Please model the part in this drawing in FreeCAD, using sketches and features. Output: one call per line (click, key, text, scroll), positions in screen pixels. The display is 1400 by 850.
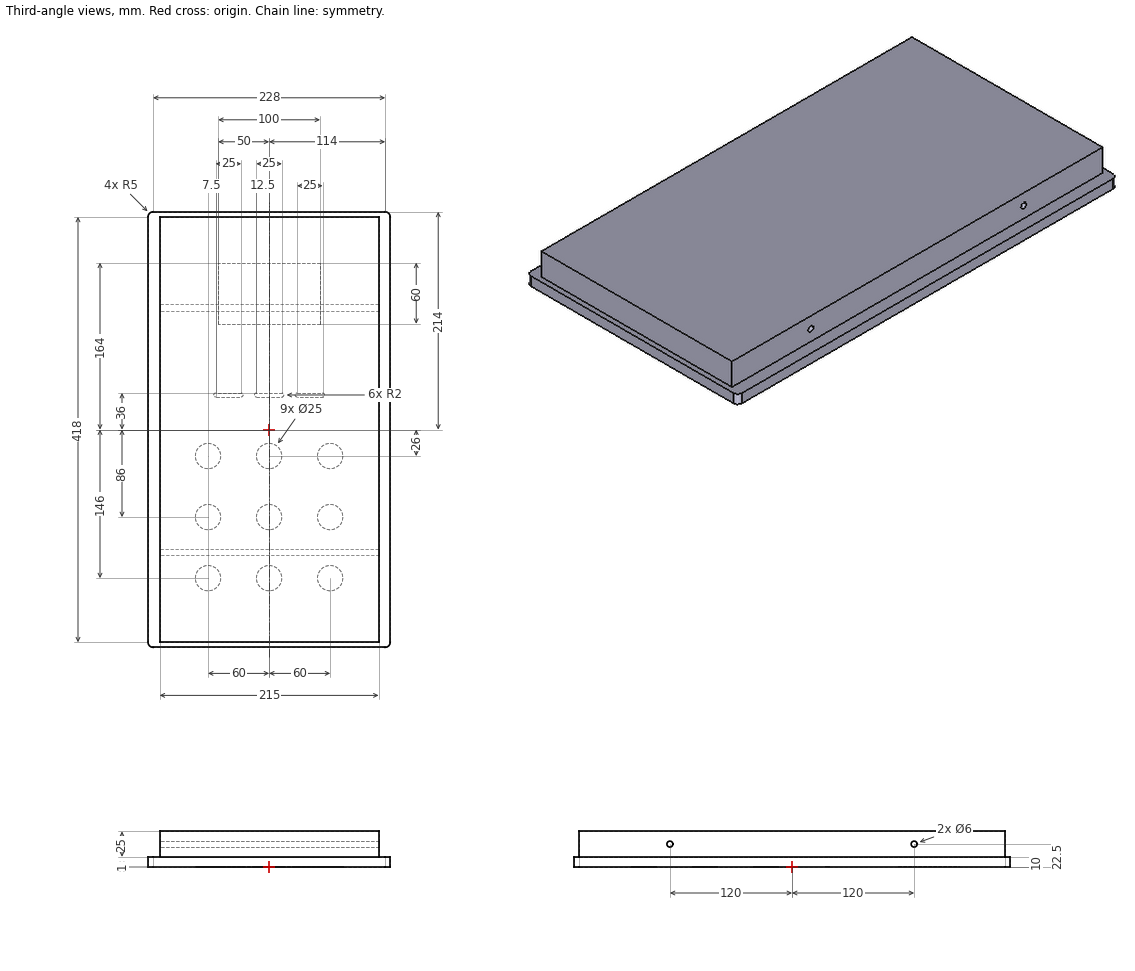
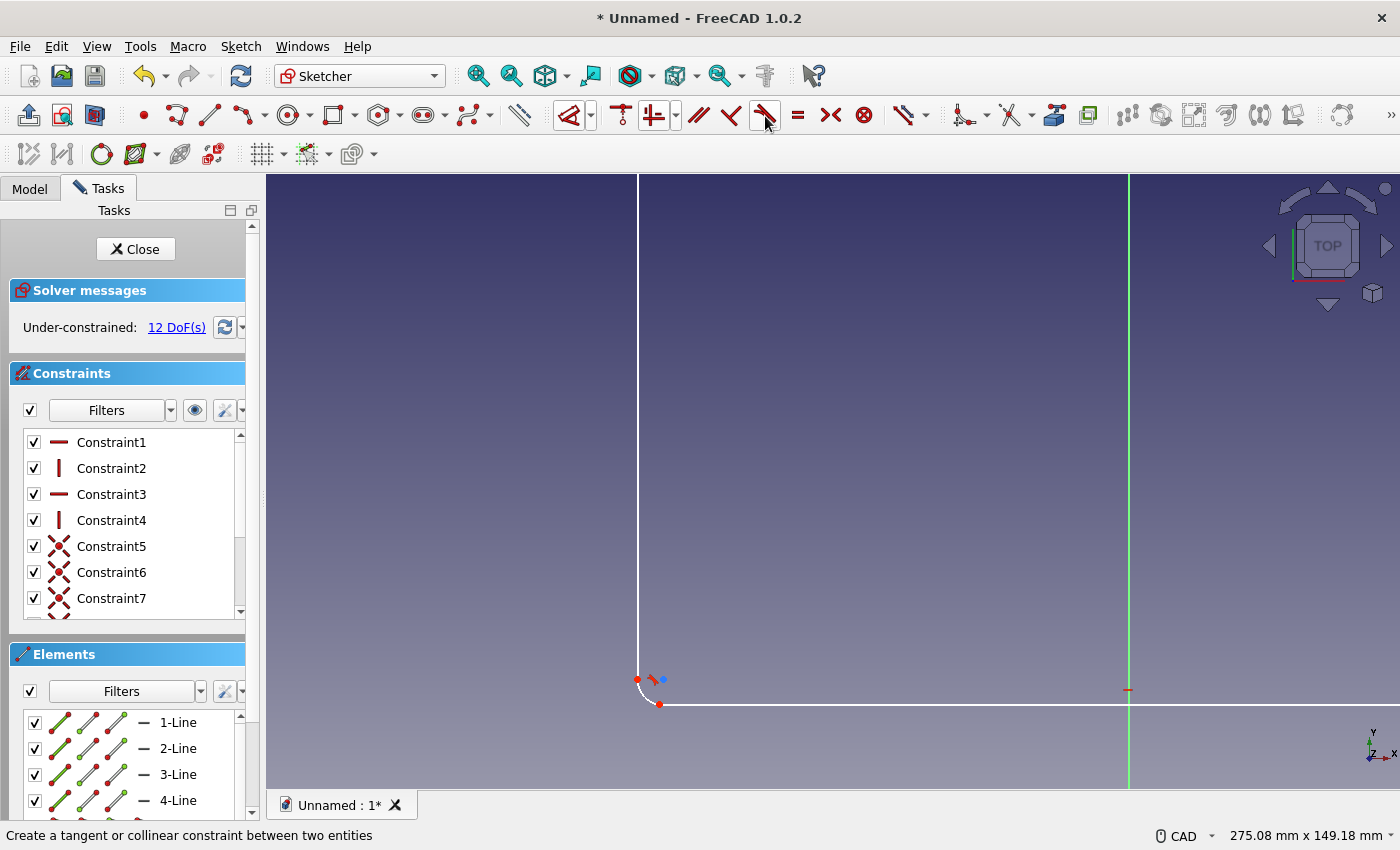
scroll(645, 698, down, 7)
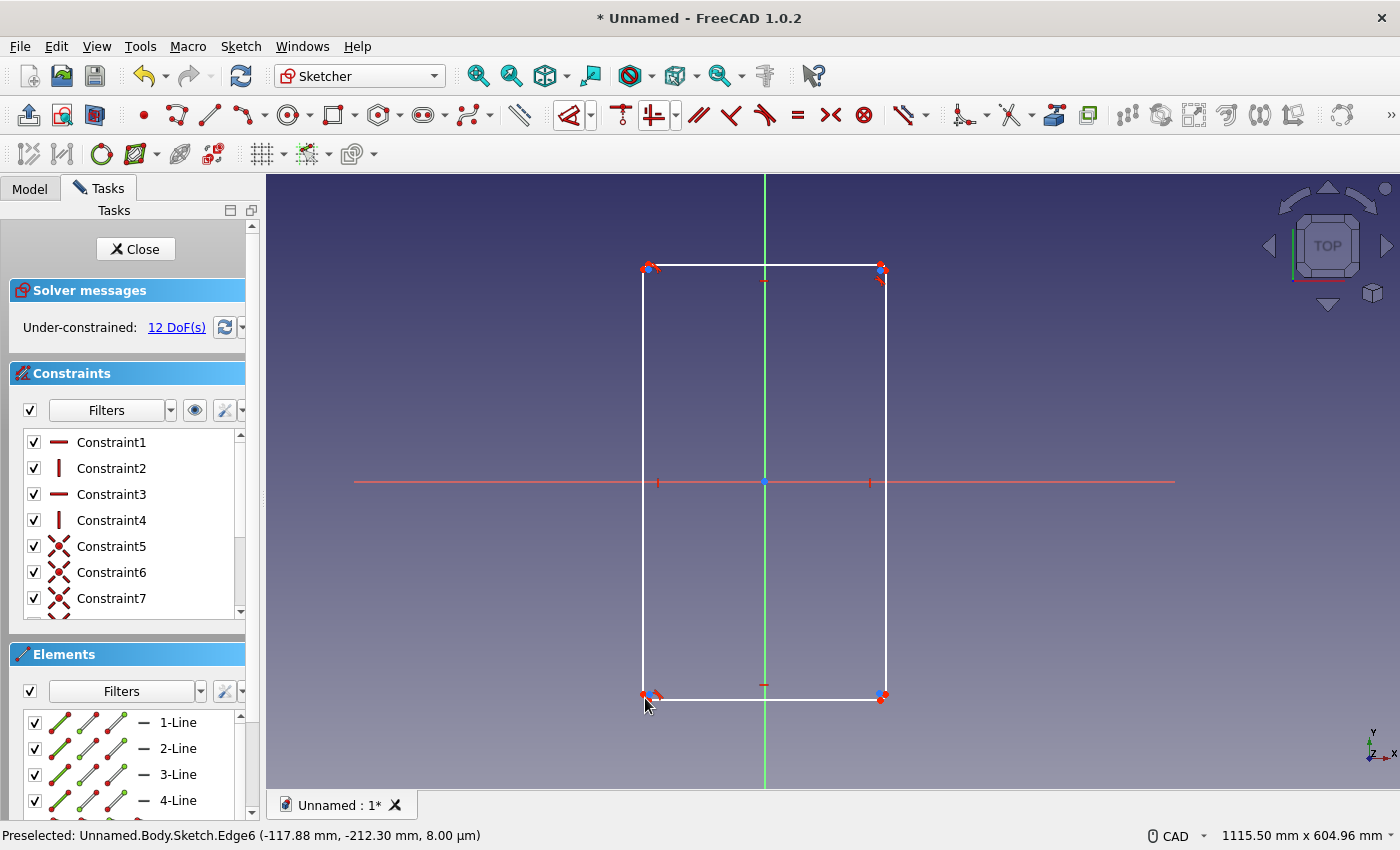
click(718, 700)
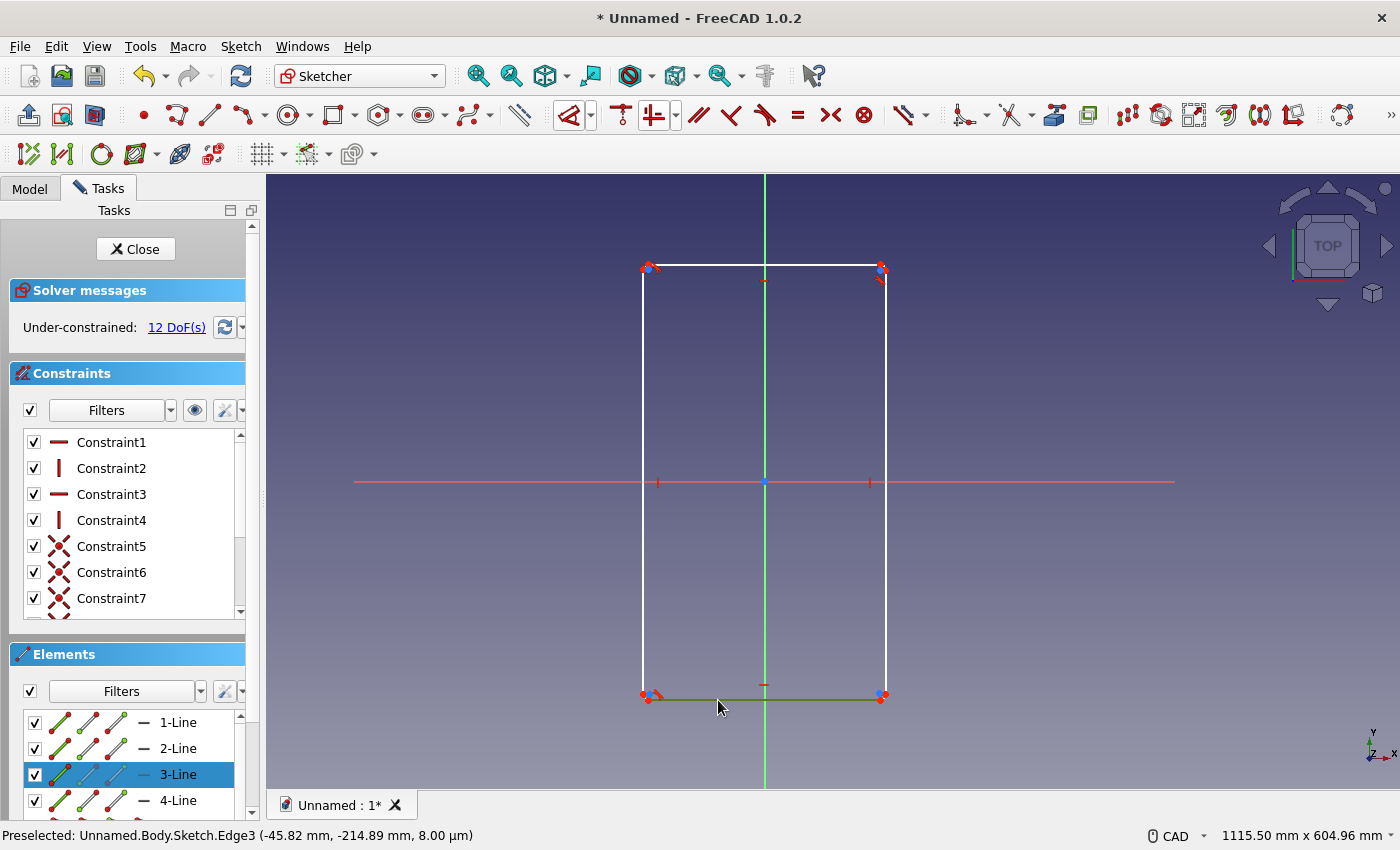
scroll(645, 698, up, 6)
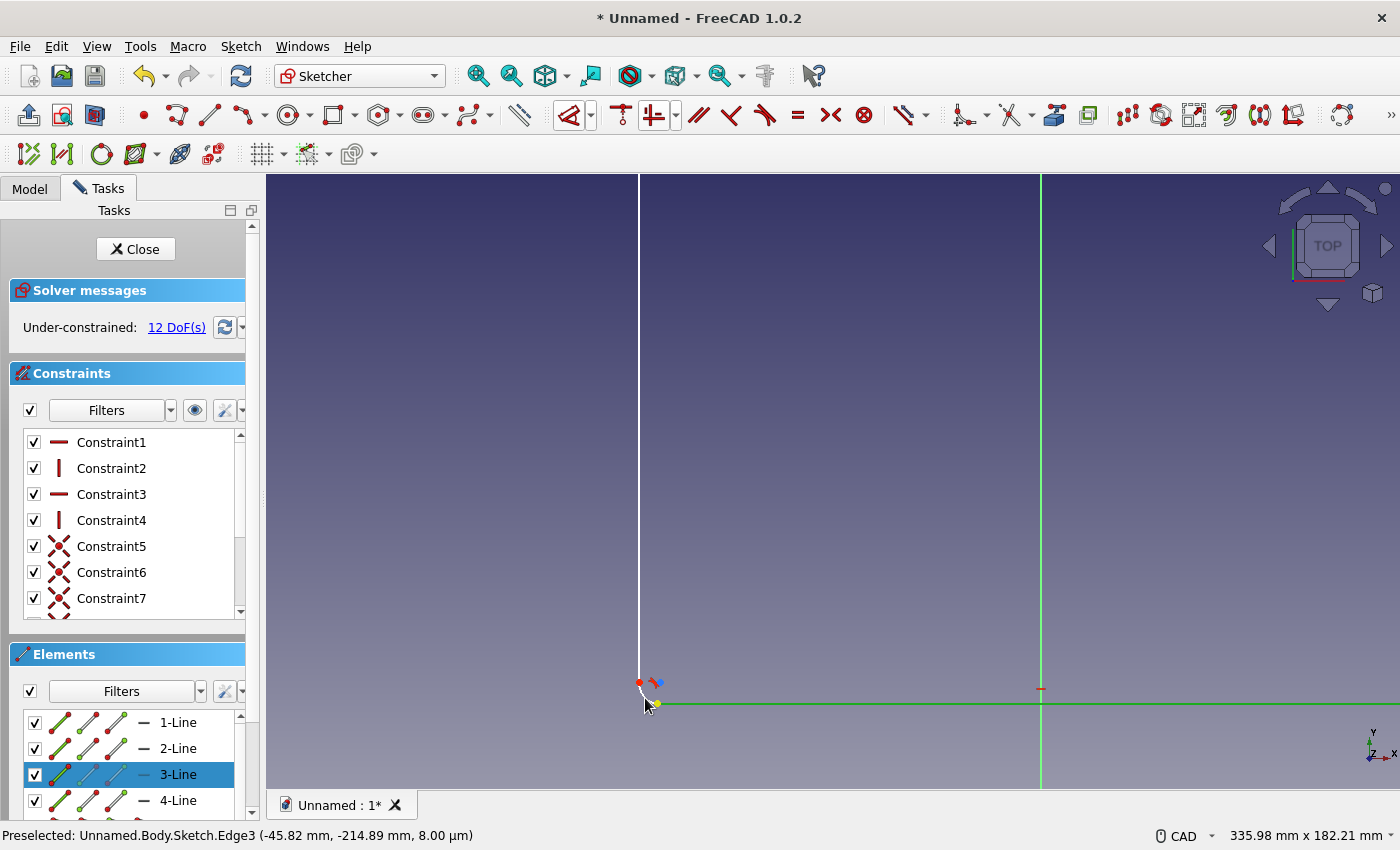
click(644, 697)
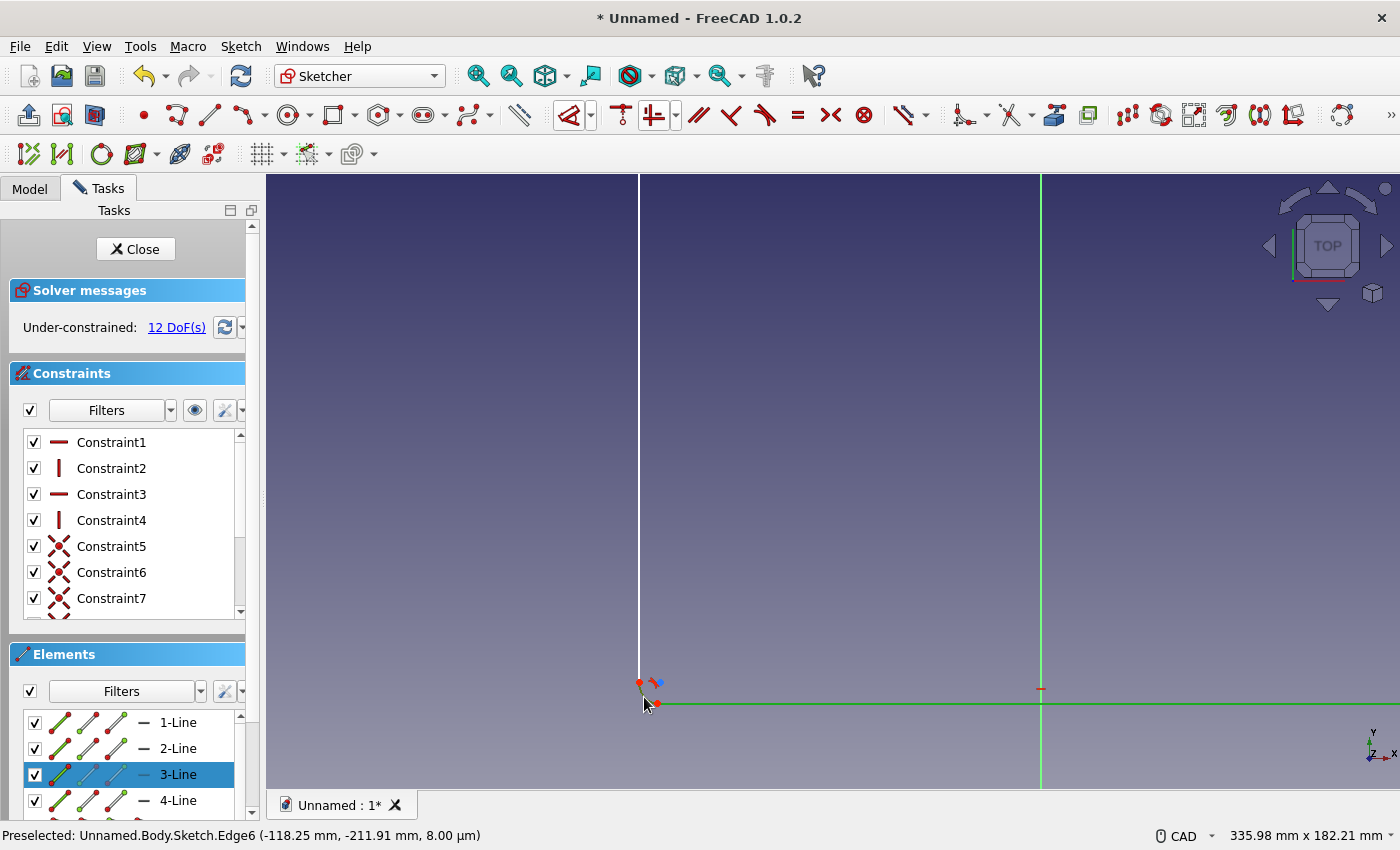
click(765, 116)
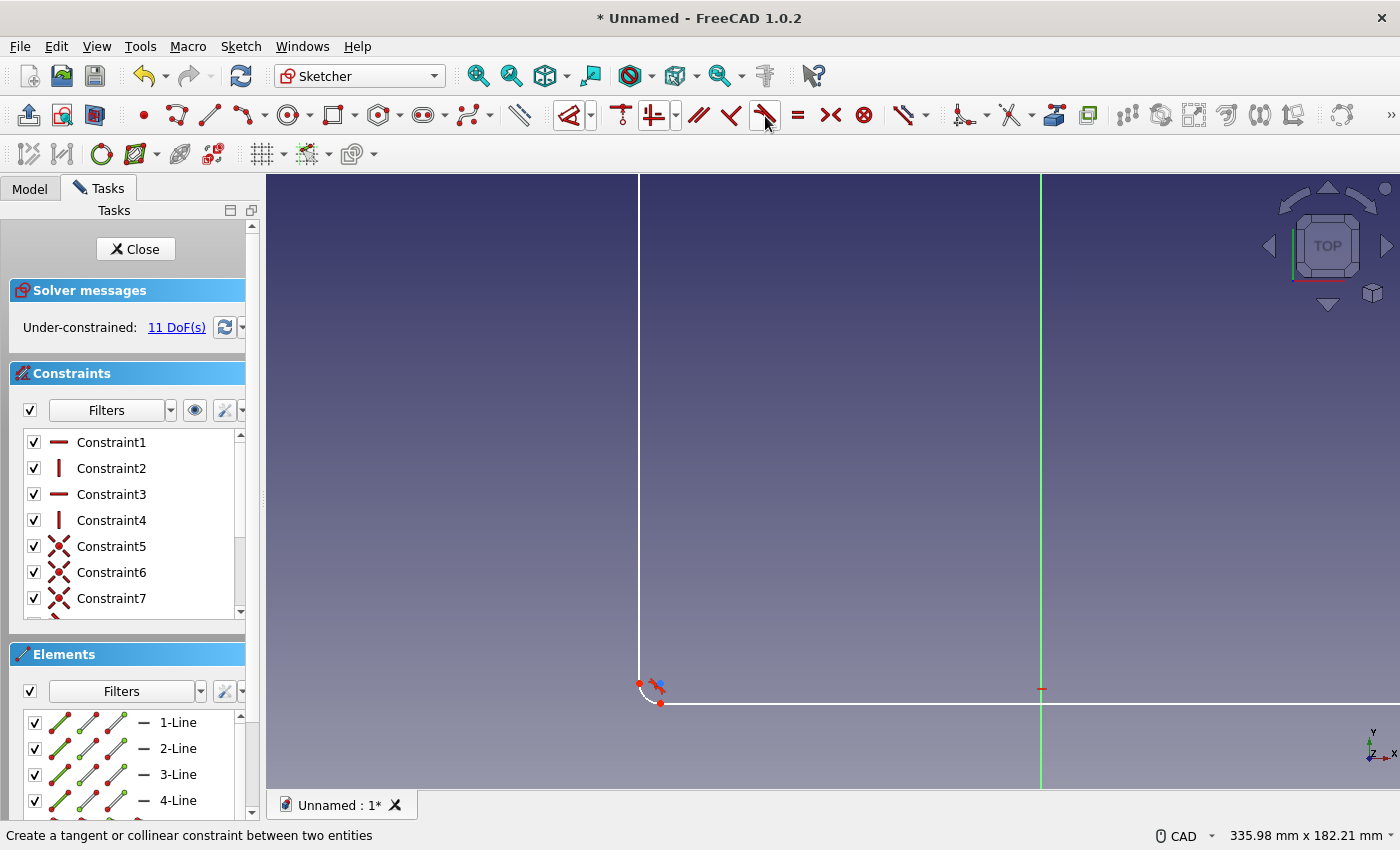
click(890, 704)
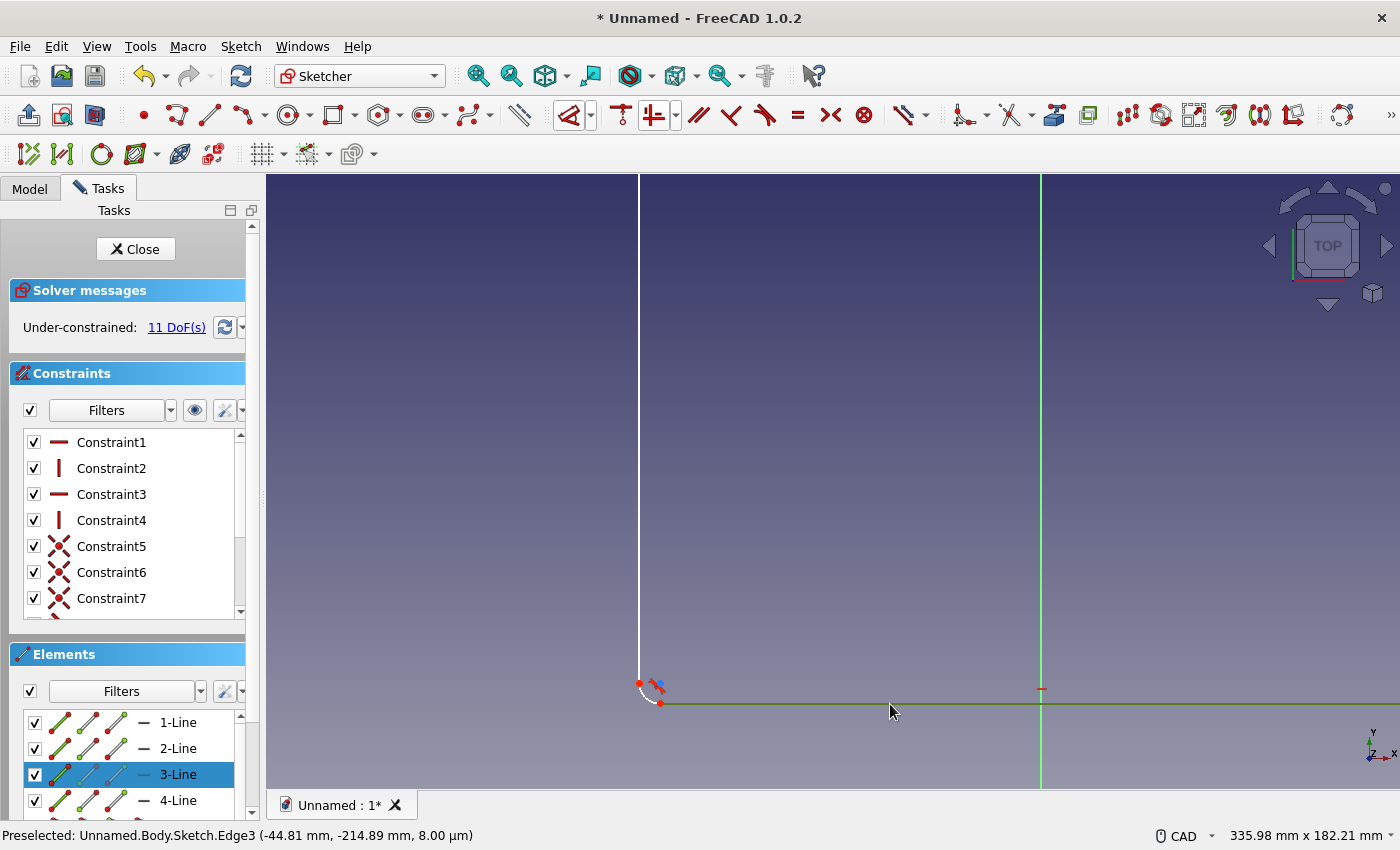
scroll(645, 698, down, 6)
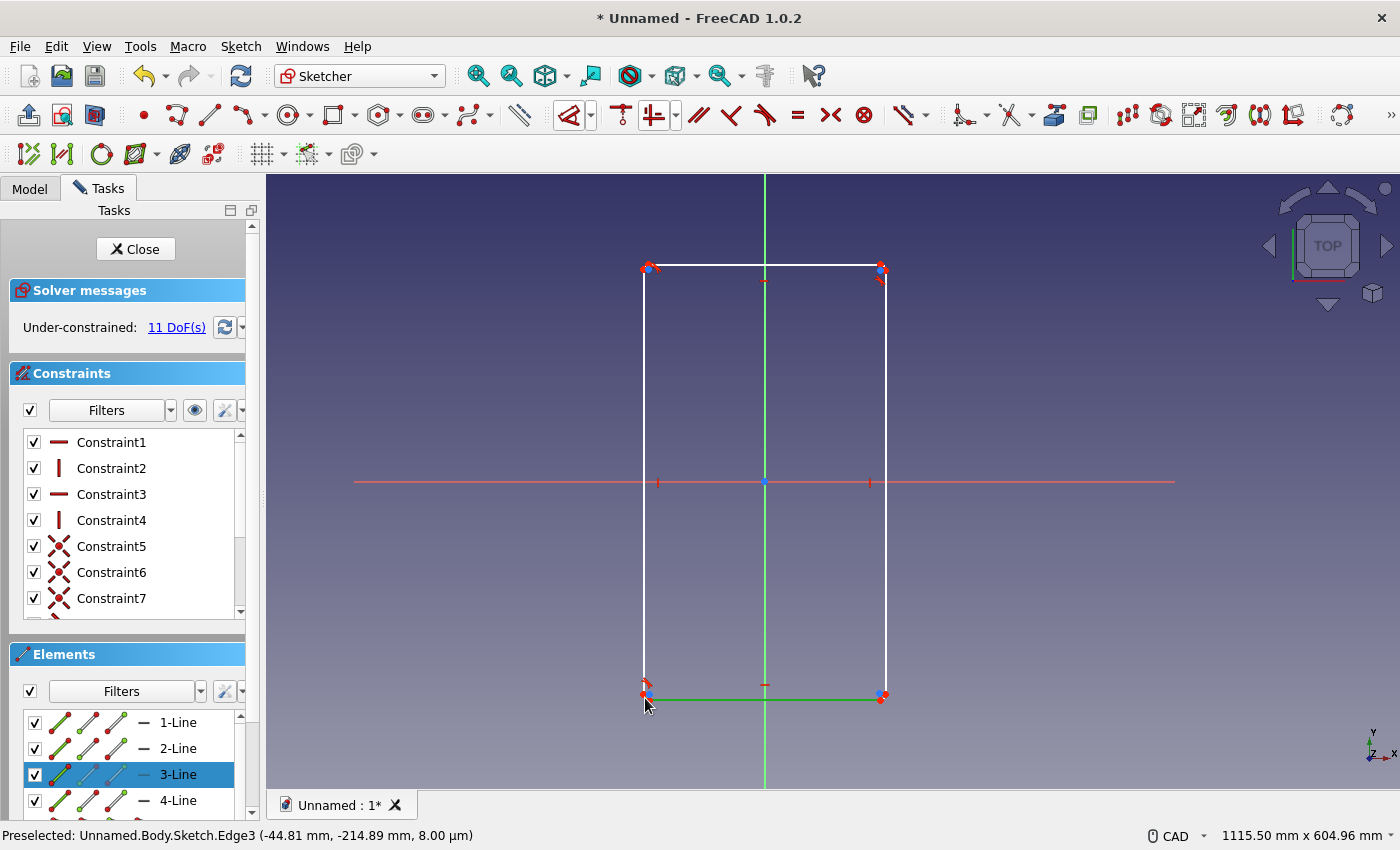
scroll(884, 698, up, 6)